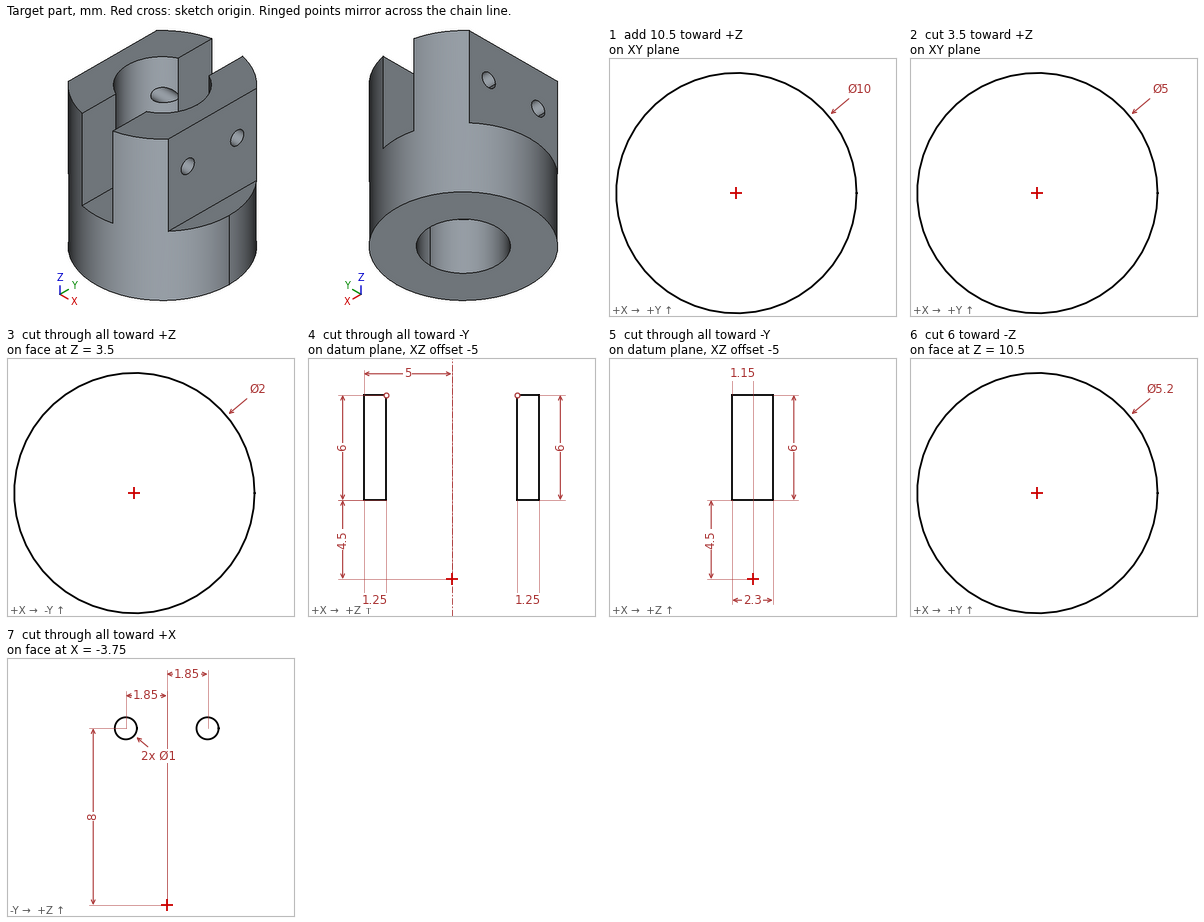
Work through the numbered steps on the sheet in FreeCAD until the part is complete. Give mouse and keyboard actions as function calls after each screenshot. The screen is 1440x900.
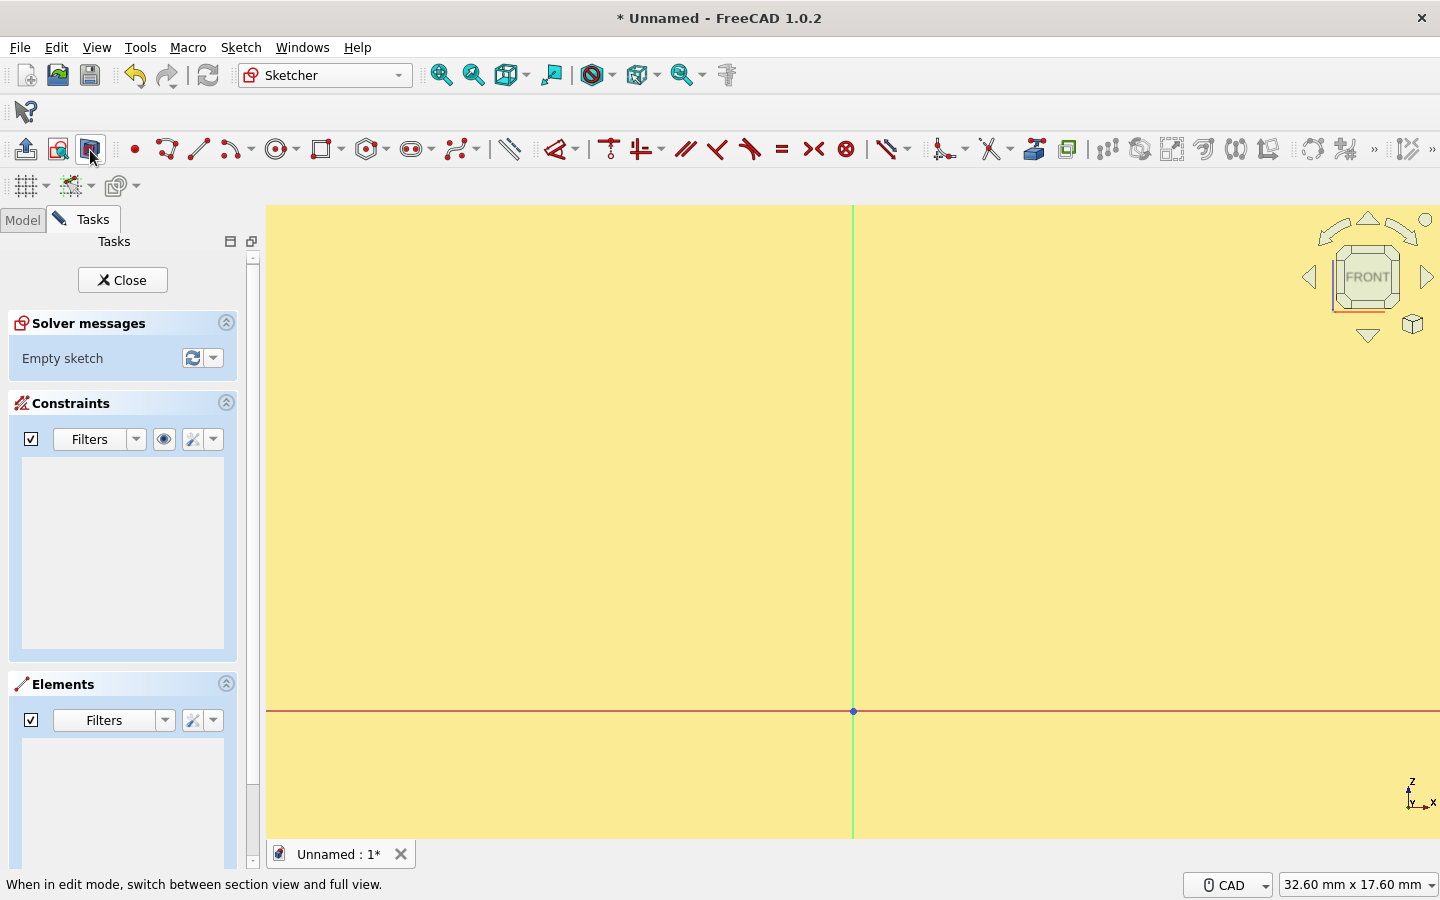
key(g)
key(r)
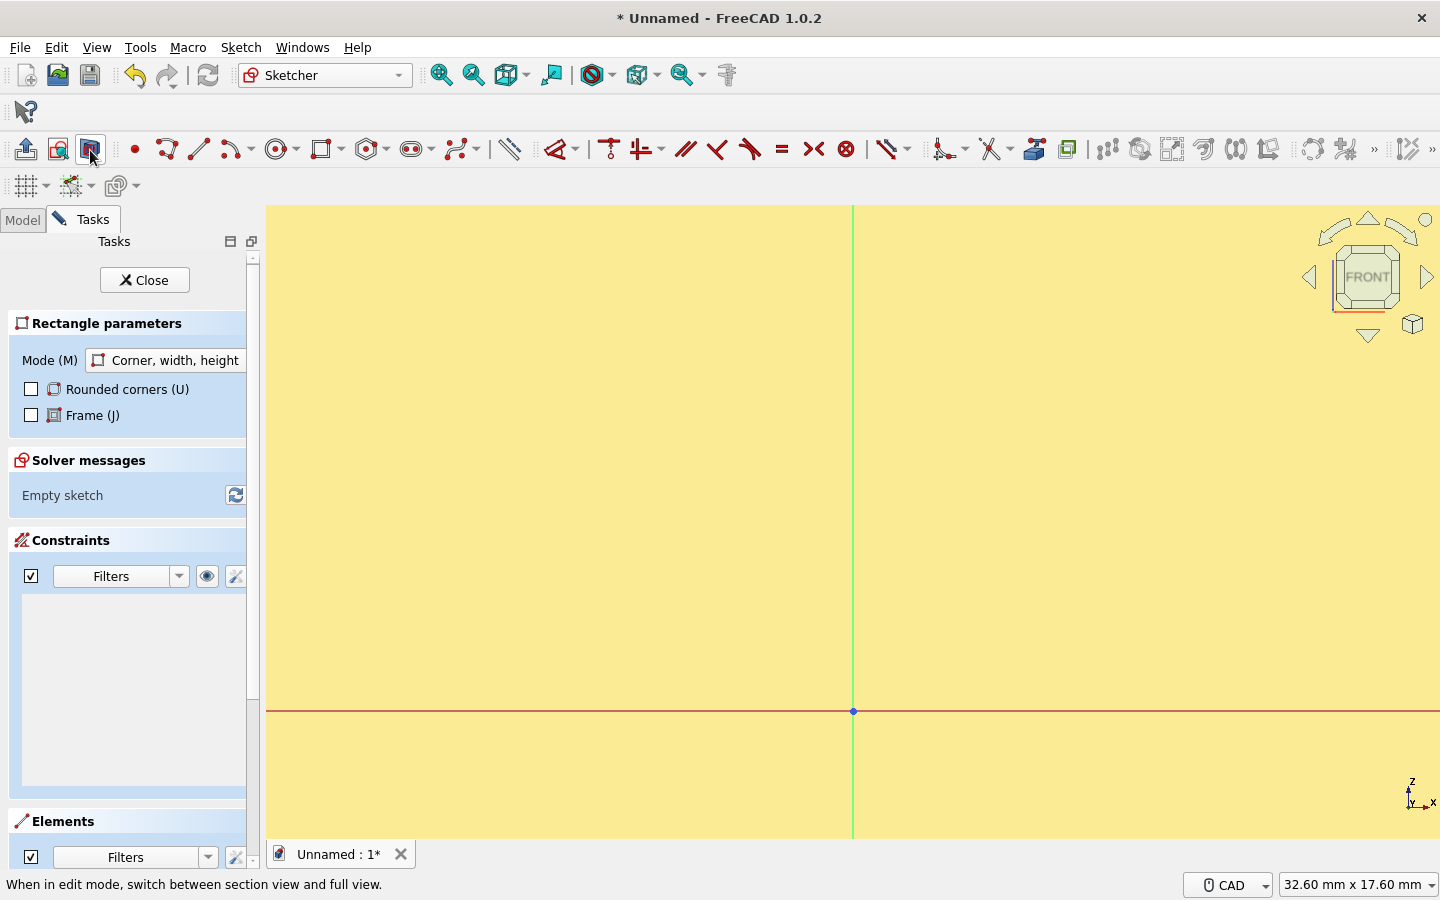
click(673, 333)
move(718, 549)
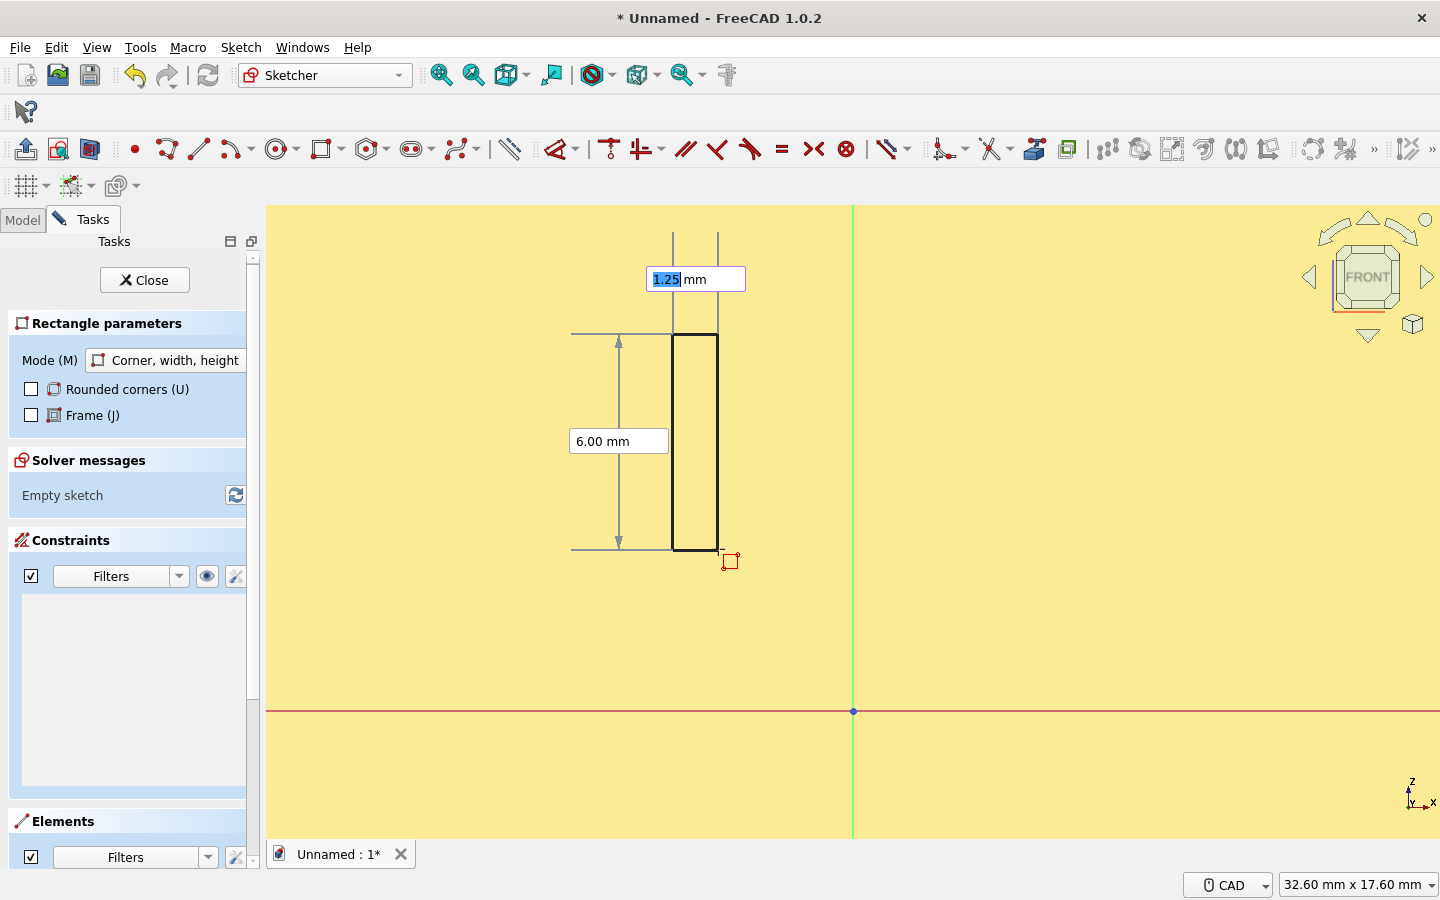
text(1.25)
key(Tab)
text(6)
key(Return)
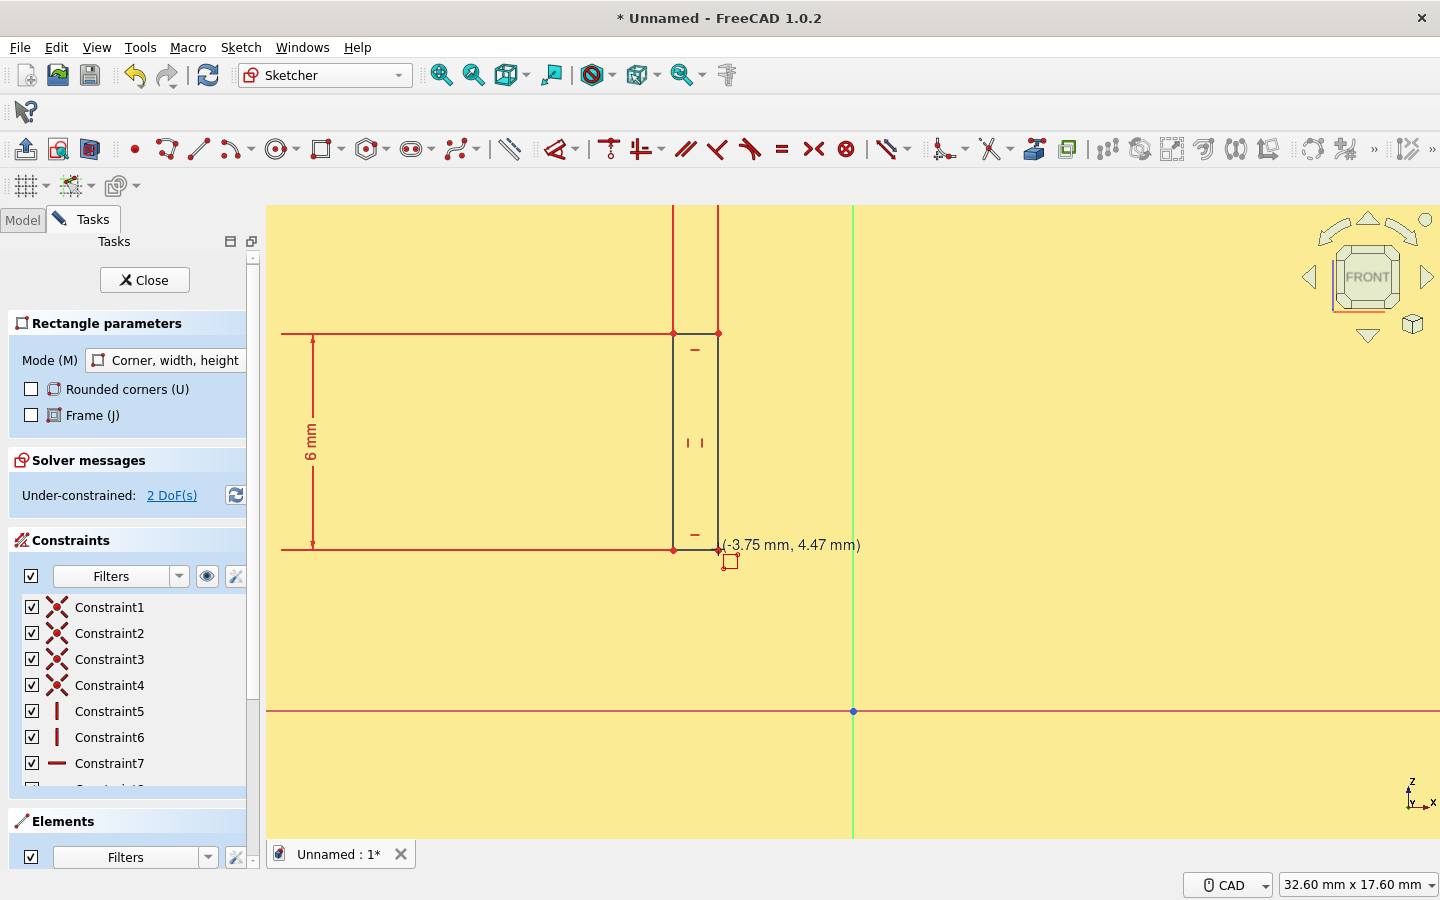
click(988, 333)
move(1033, 549)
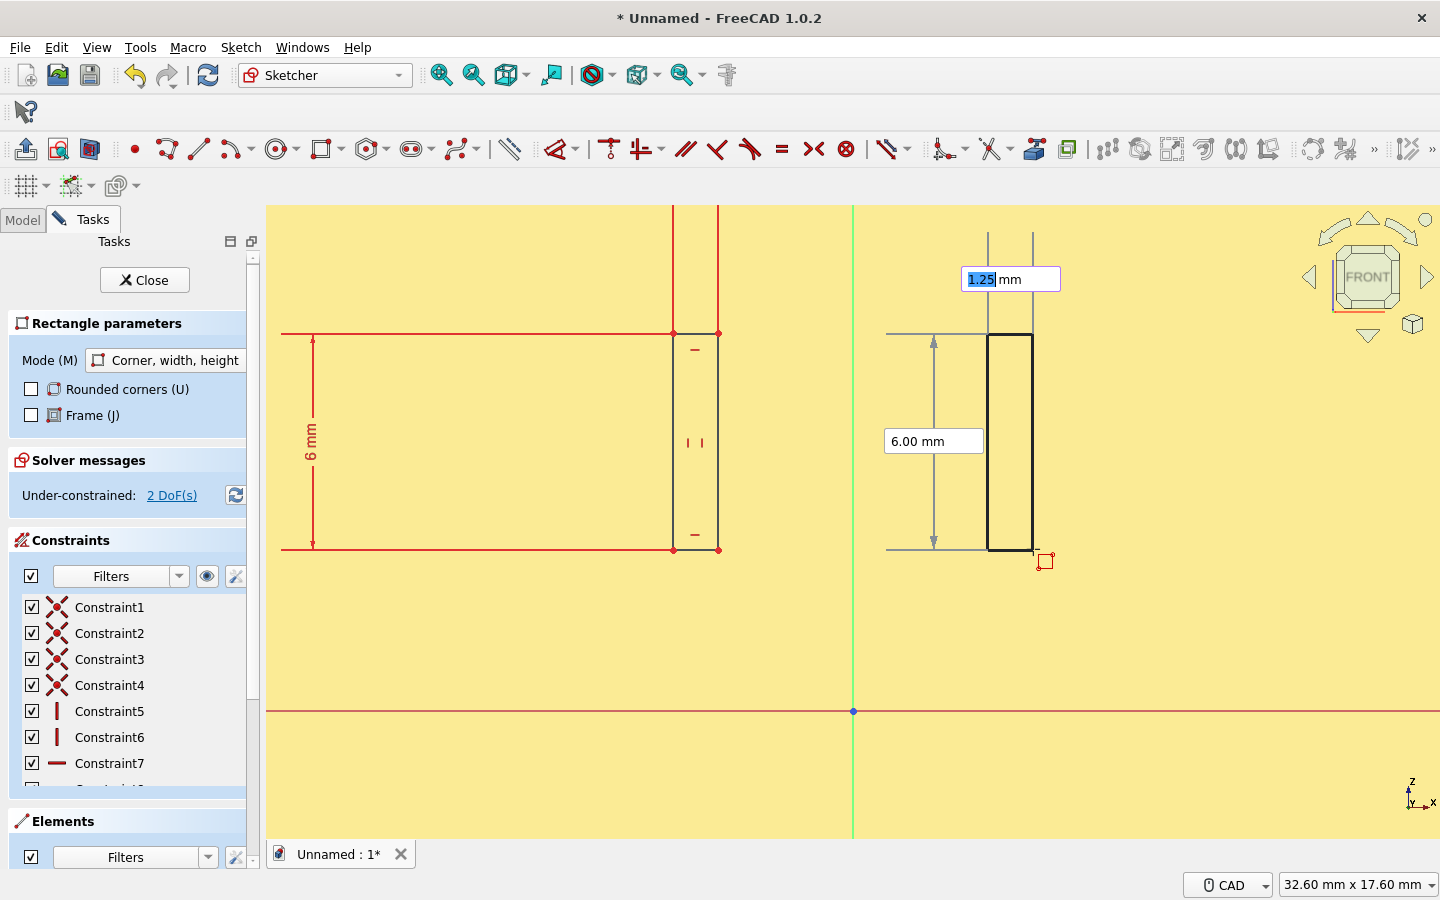
text(1.25)
key(Tab)
text(6)
key(Return)
key(Escape)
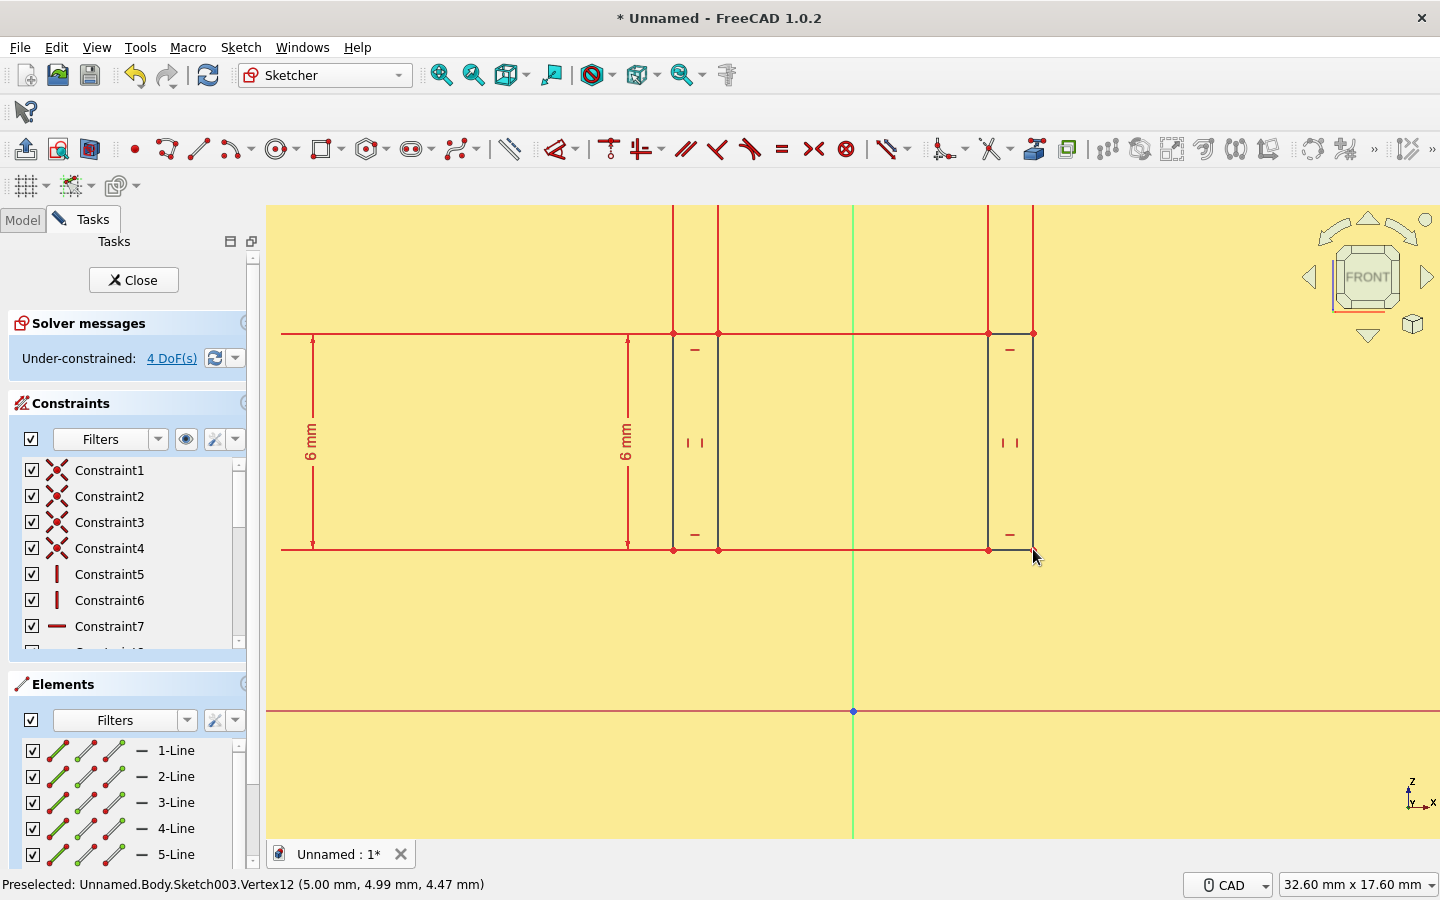
click(718, 334)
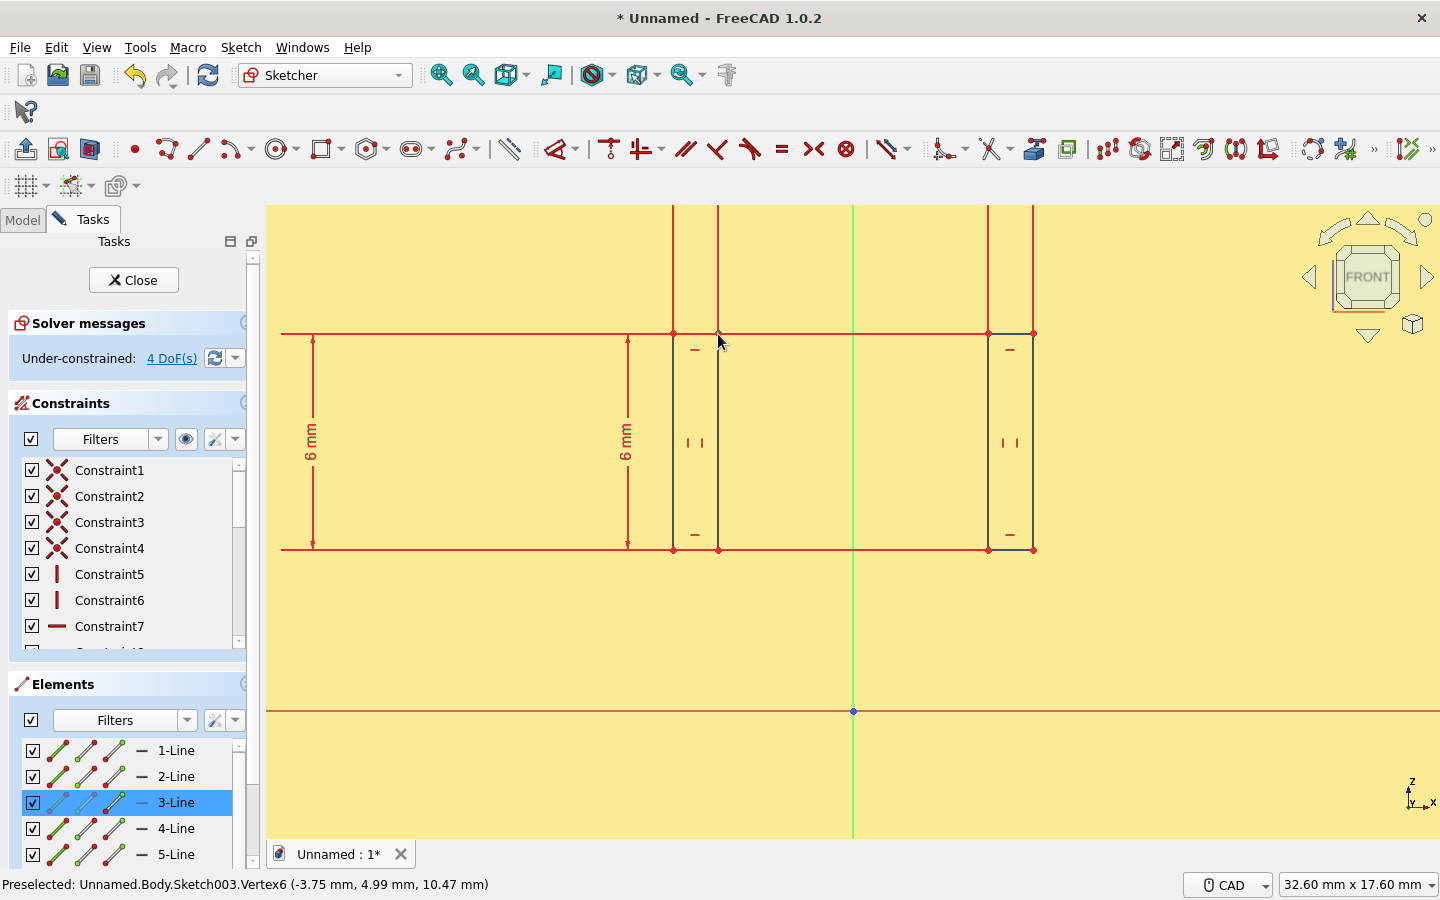
click(988, 334)